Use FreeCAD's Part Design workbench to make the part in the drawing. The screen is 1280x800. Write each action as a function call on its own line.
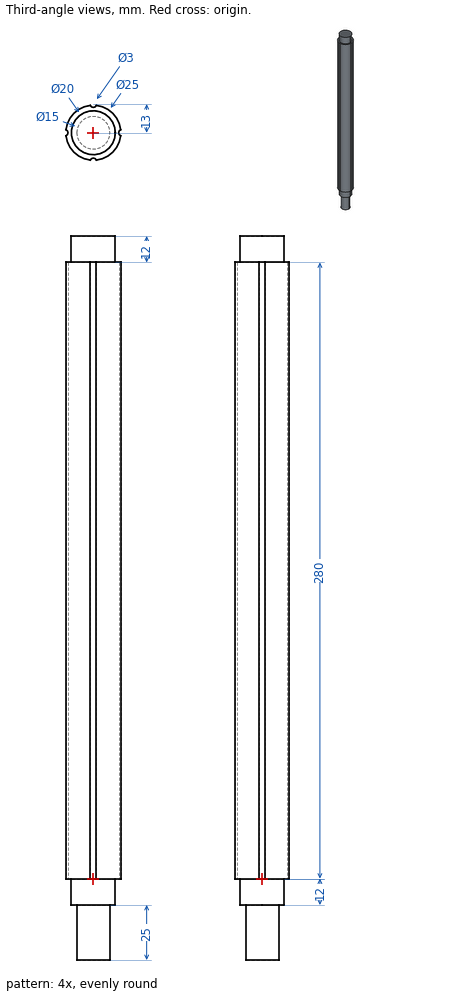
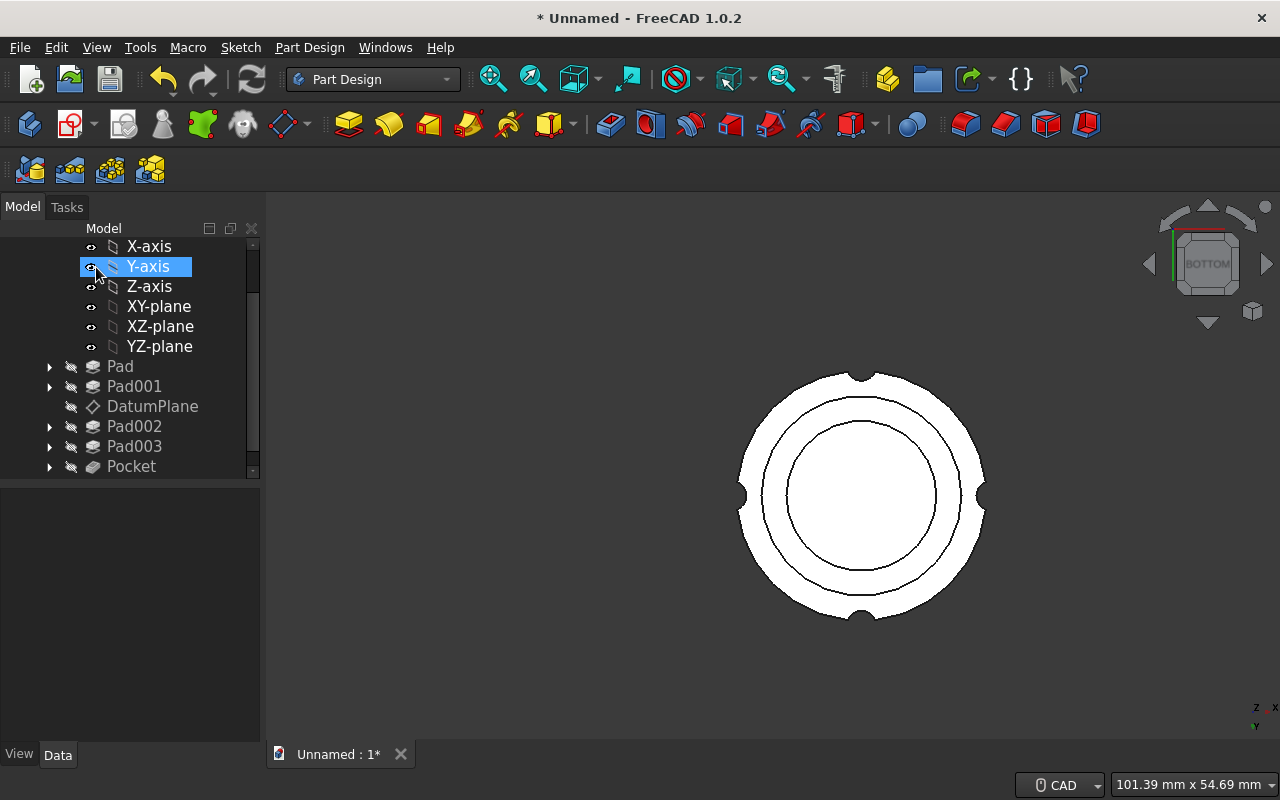
key(0)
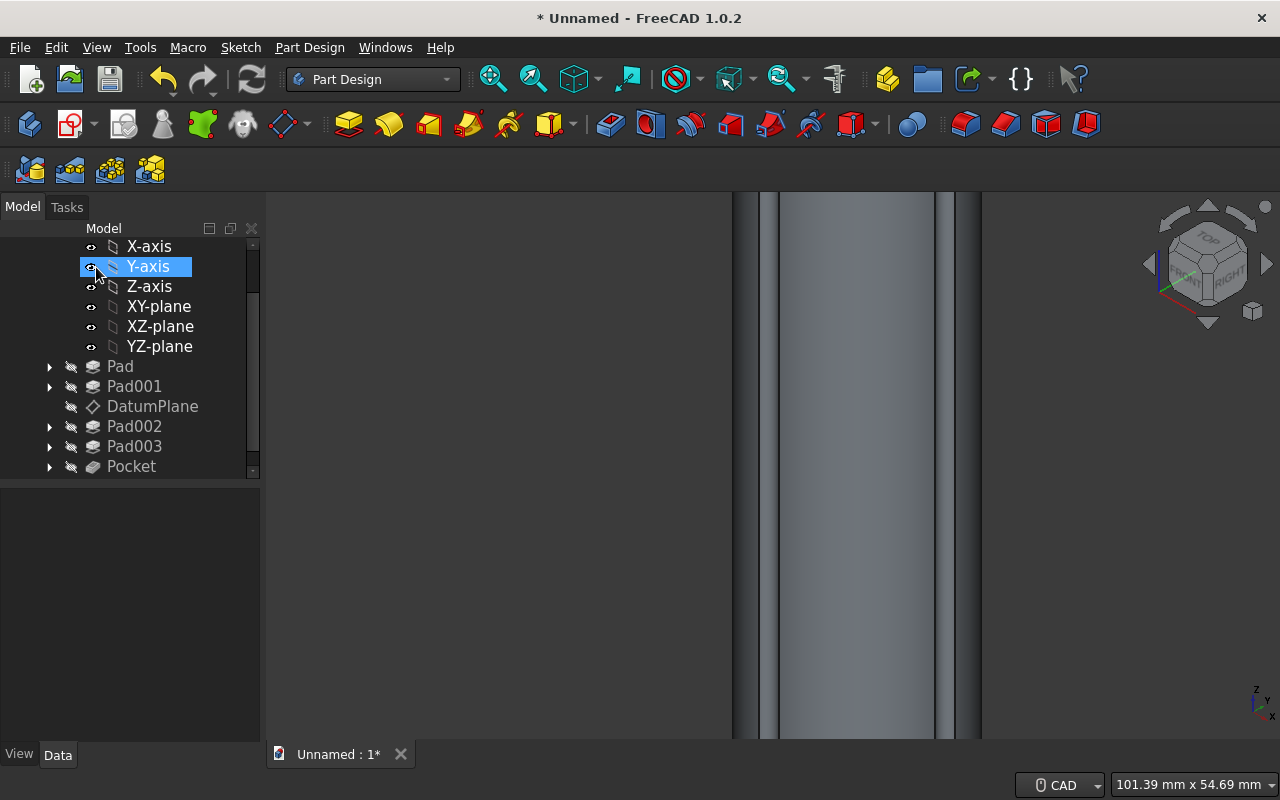
key(v)
key(f)